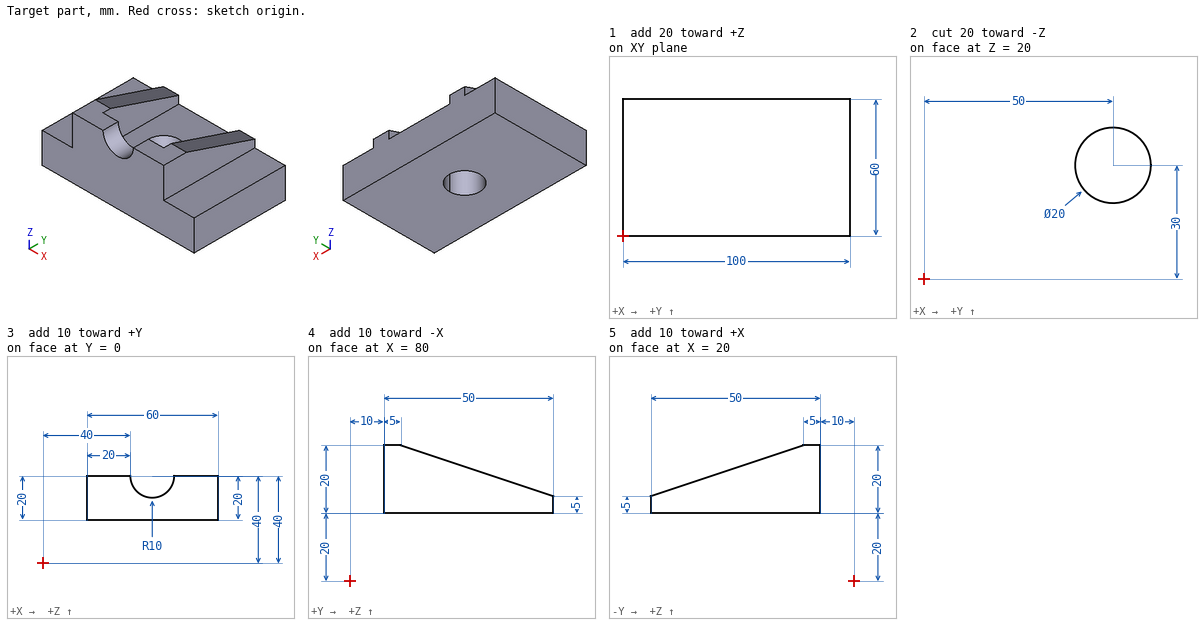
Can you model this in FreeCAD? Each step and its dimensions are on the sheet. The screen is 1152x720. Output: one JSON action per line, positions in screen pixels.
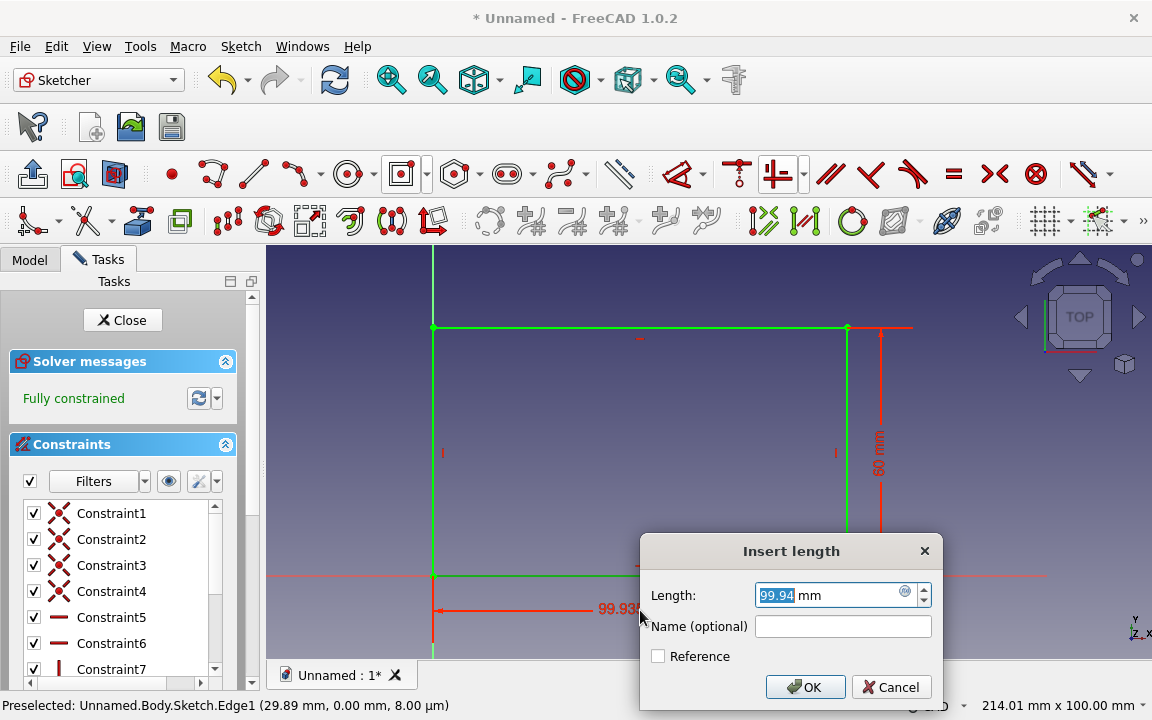
{"action": "type", "text": "100"}
{"action": "key", "text": "Return"}
{"action": "key", "text": "Escape"}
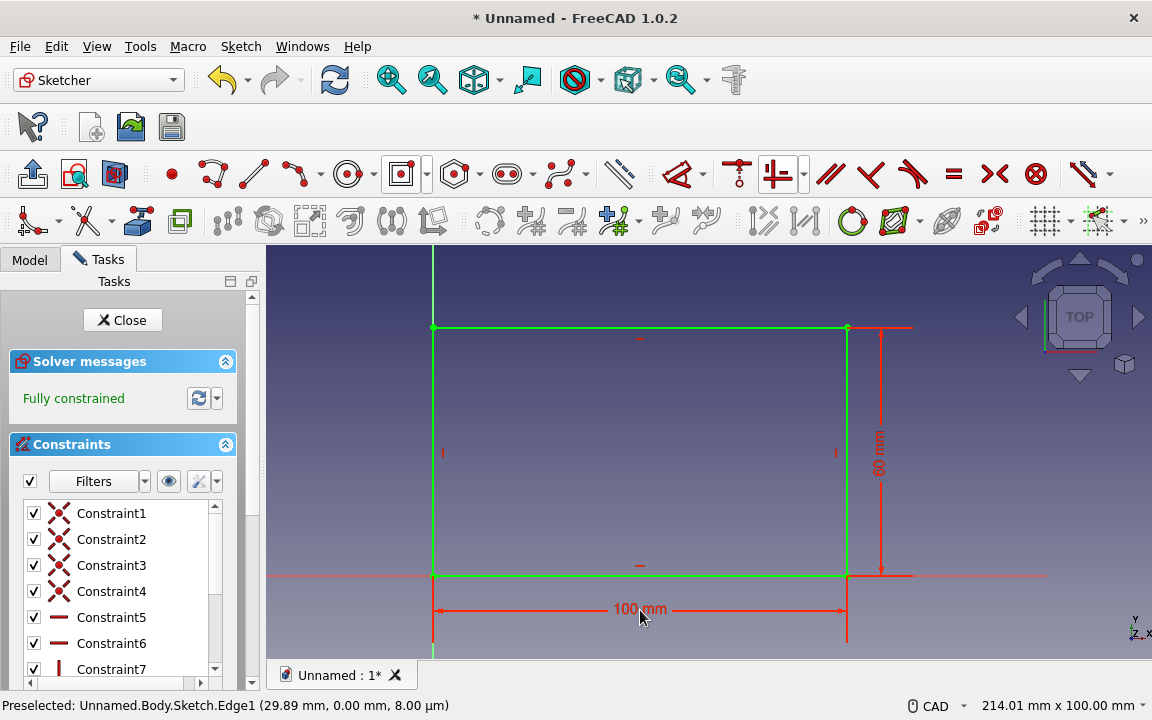
{"action": "left_click", "coordinate": [123, 320]}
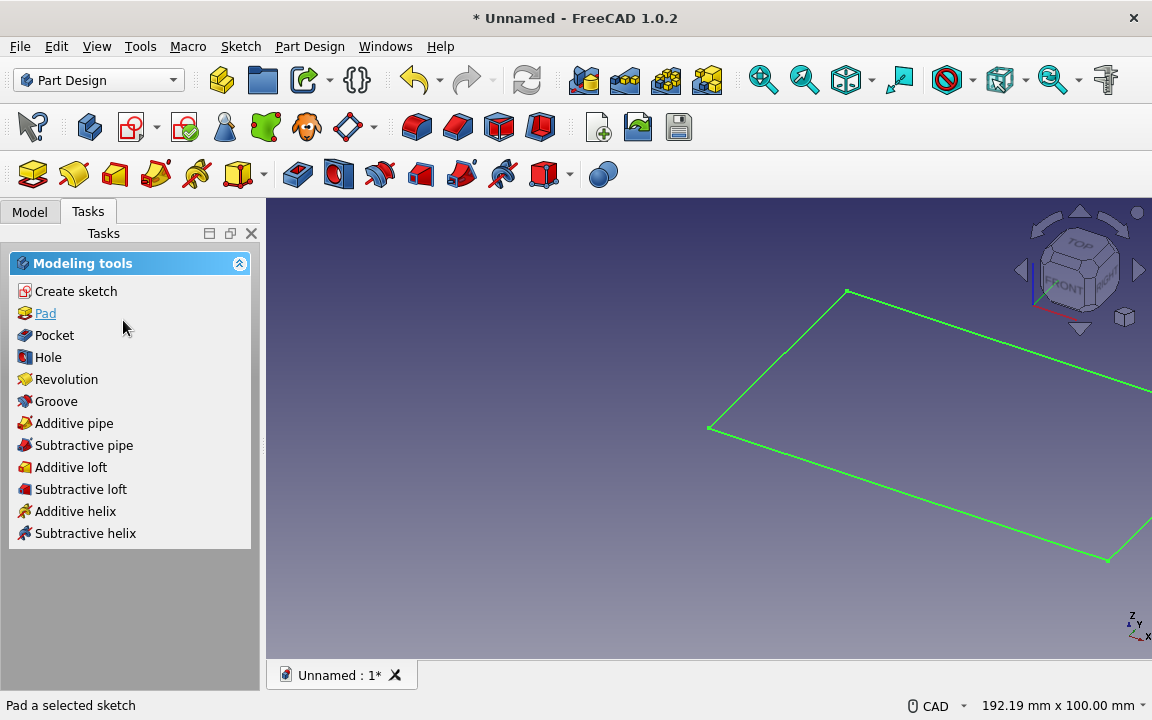
{"action": "left_click", "coordinate": [33, 174]}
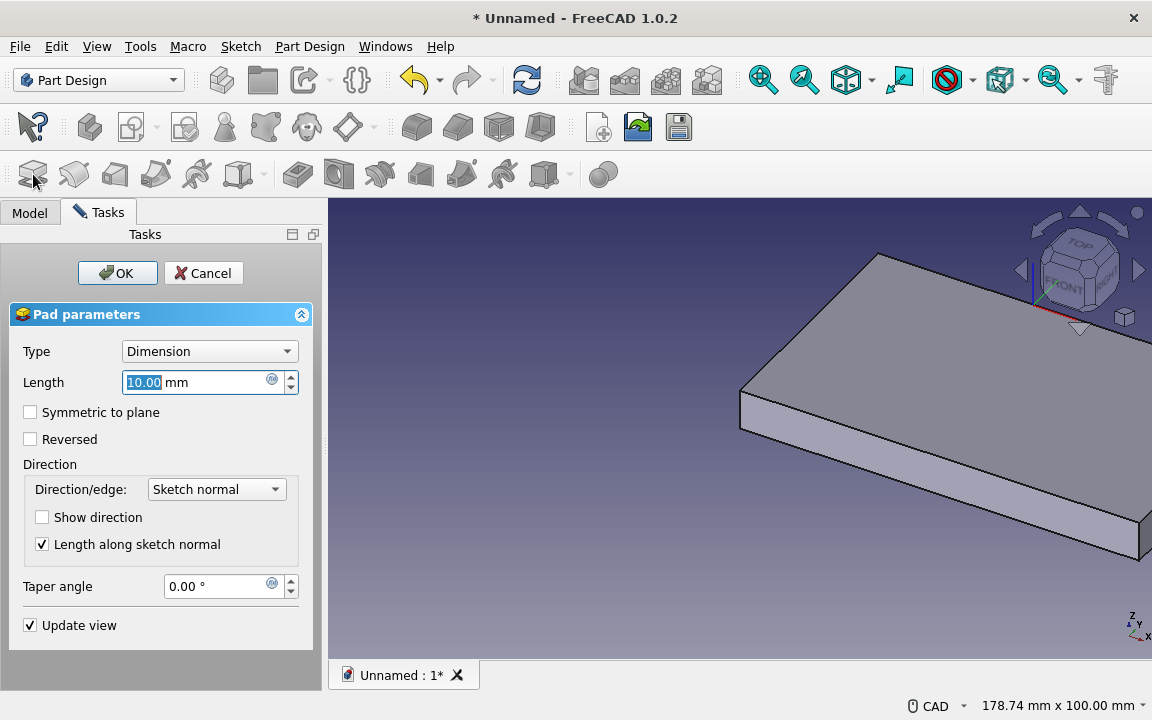
{"action": "type", "text": "20"}
{"action": "key", "text": "Tab"}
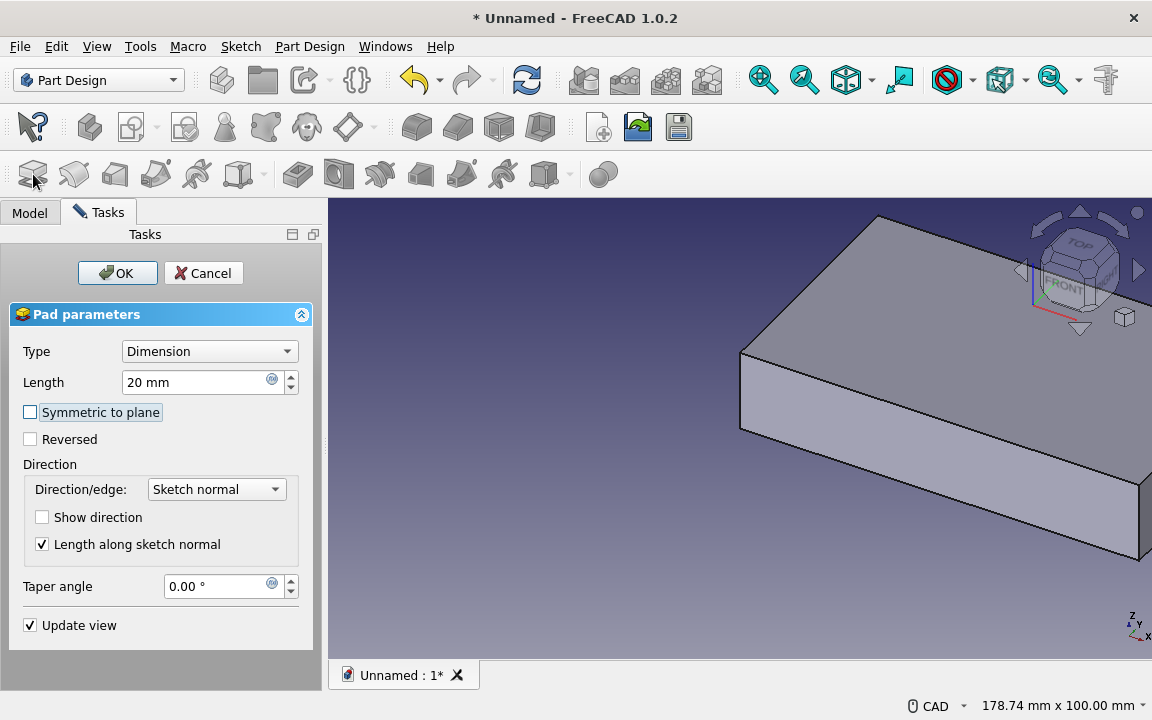
{"action": "left_click", "coordinate": [118, 273]}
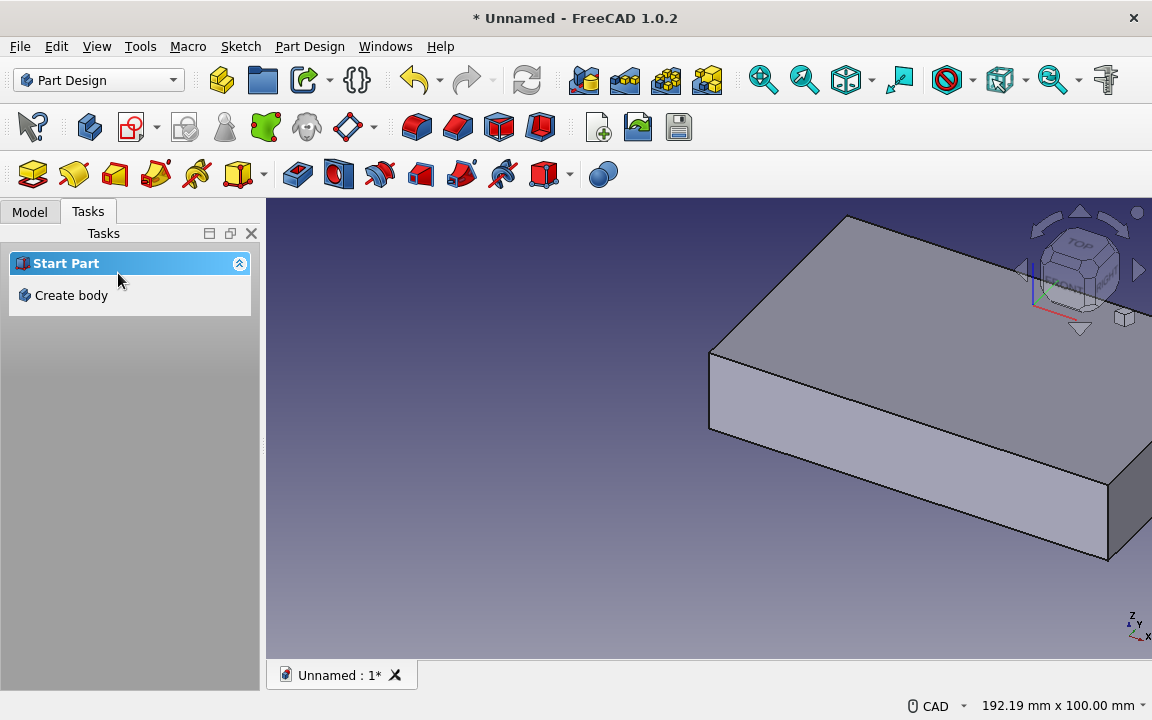
{"action": "left_click", "coordinate": [764, 80]}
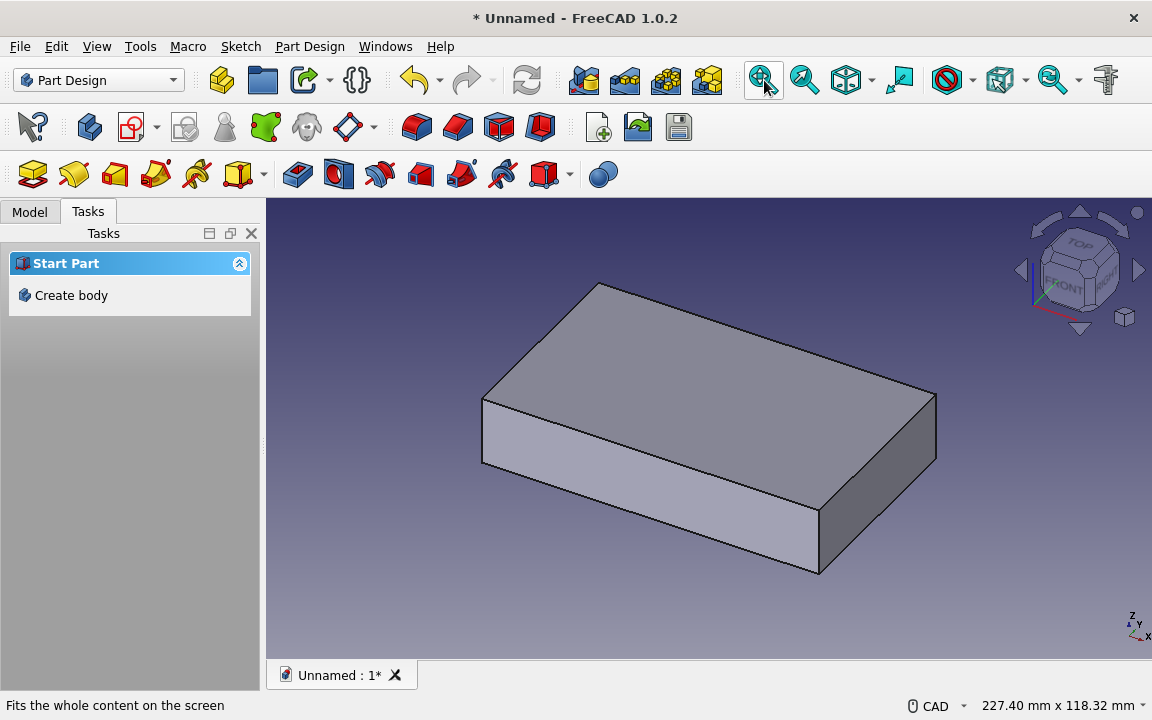
{"action": "left_click", "coordinate": [757, 412]}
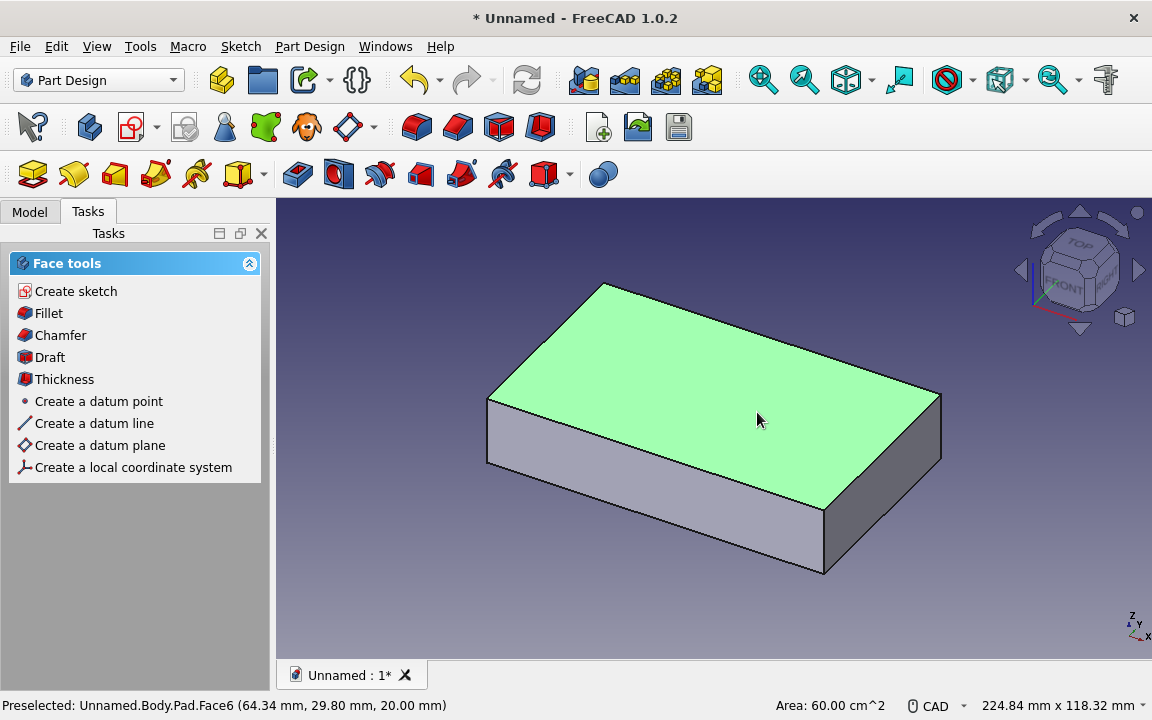
{"action": "left_click", "coordinate": [130, 128]}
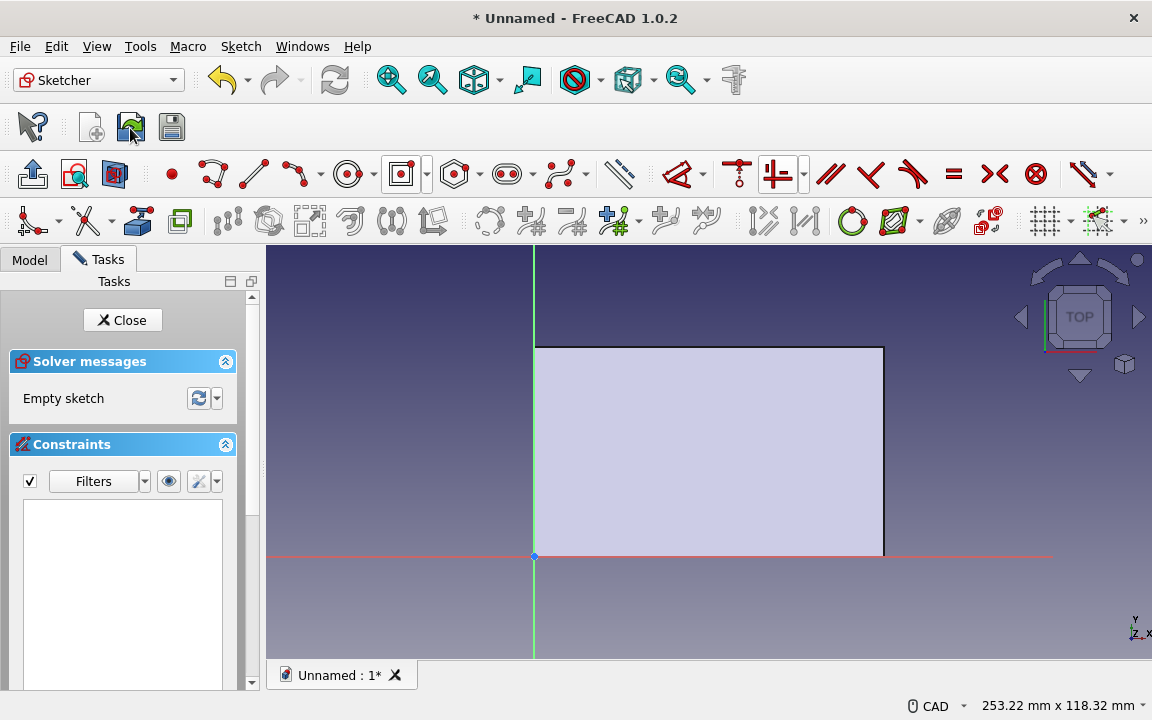
{"action": "scroll", "coordinate": [739, 452], "scroll_direction": "up", "scroll_amount": 6}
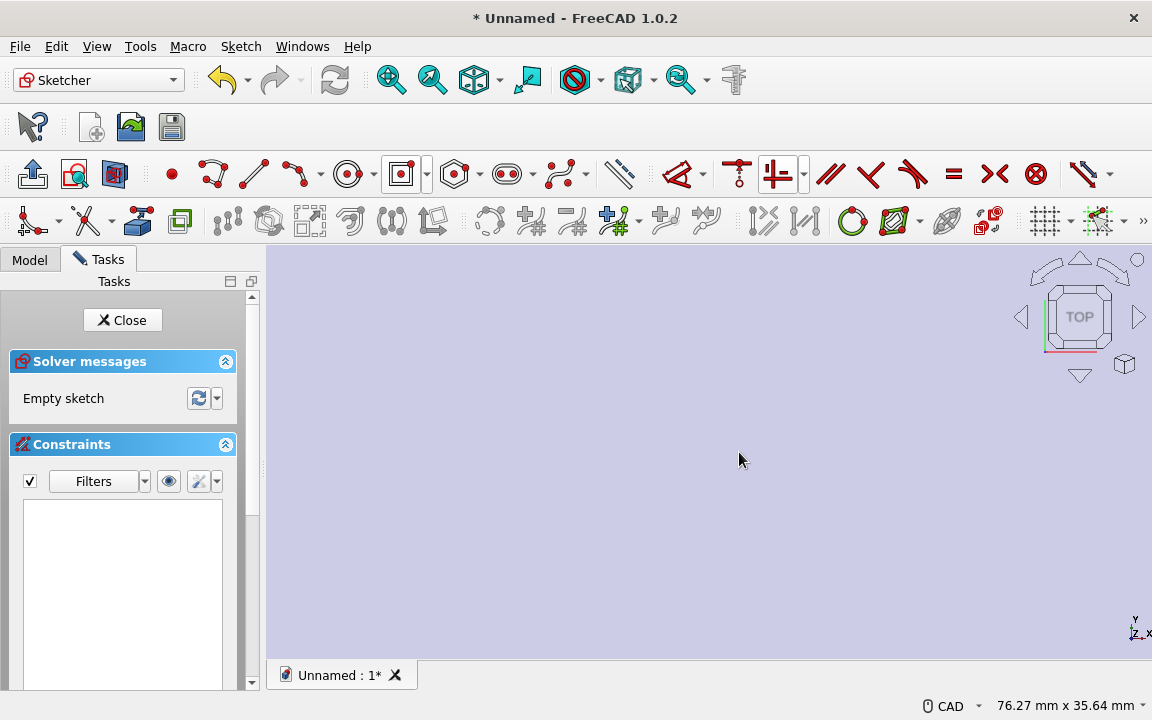
{"action": "left_click", "coordinate": [348, 174]}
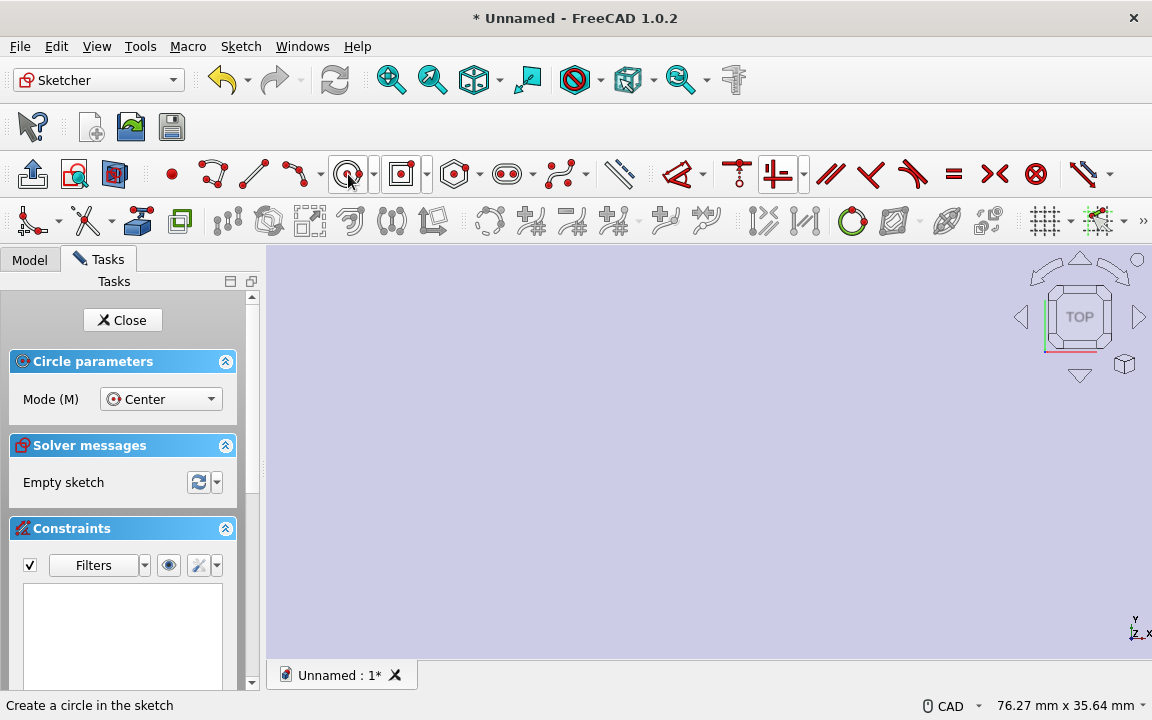
{"action": "left_click", "coordinate": [638, 451]}
{"action": "left_click", "coordinate": [720, 369]}
{"action": "key", "text": "Escape"}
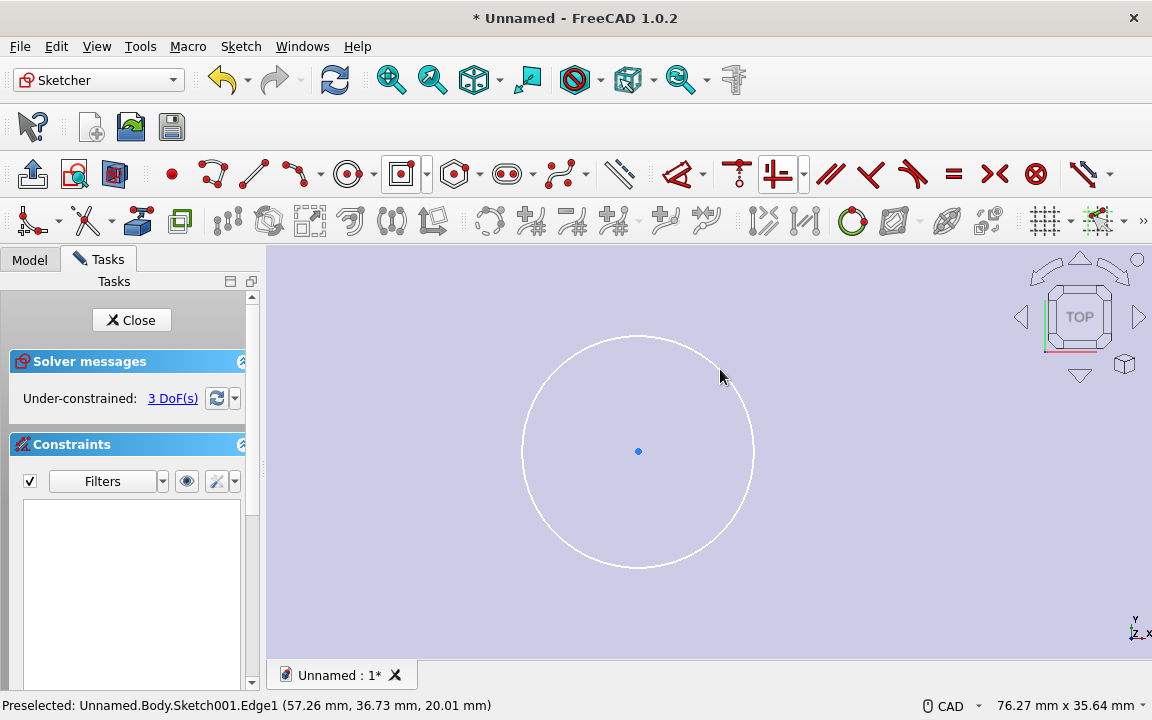
{"action": "left_click", "coordinate": [676, 174]}